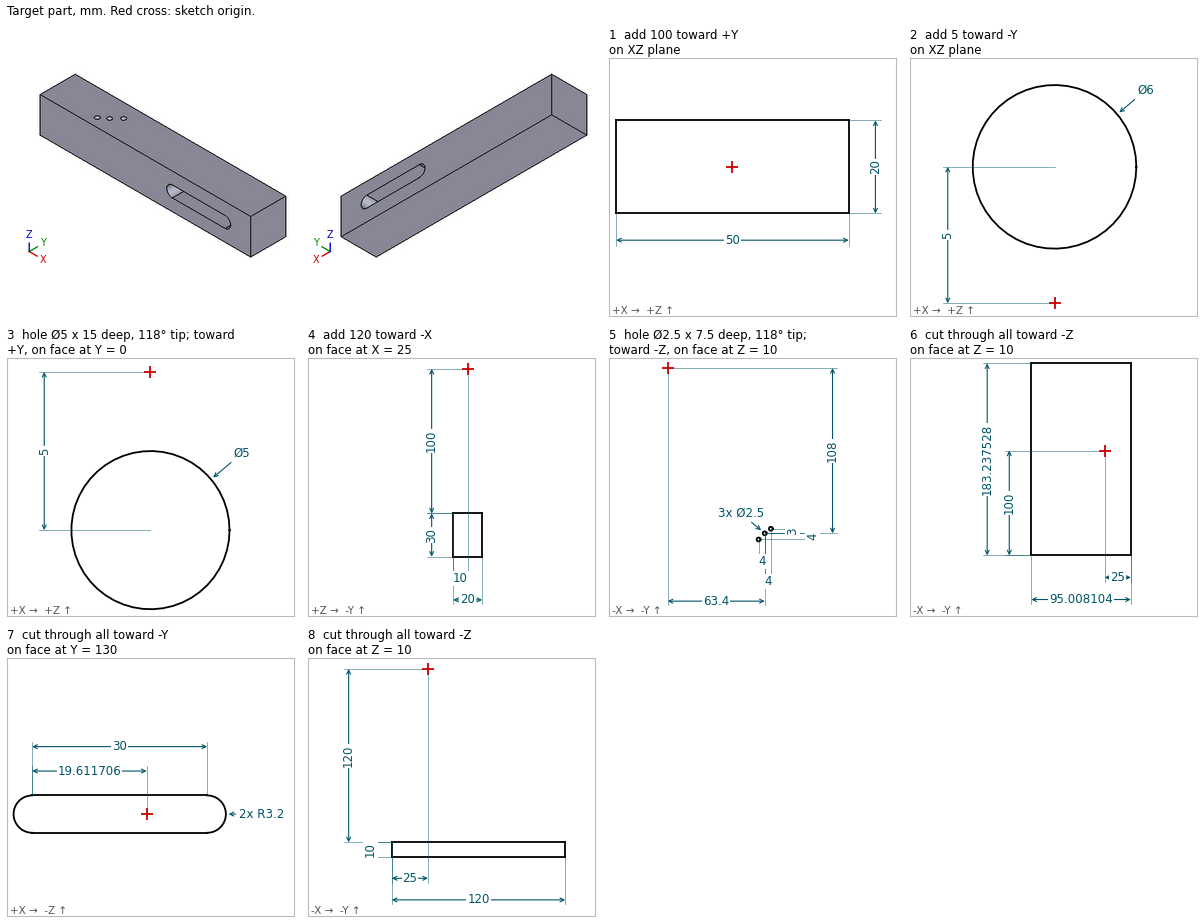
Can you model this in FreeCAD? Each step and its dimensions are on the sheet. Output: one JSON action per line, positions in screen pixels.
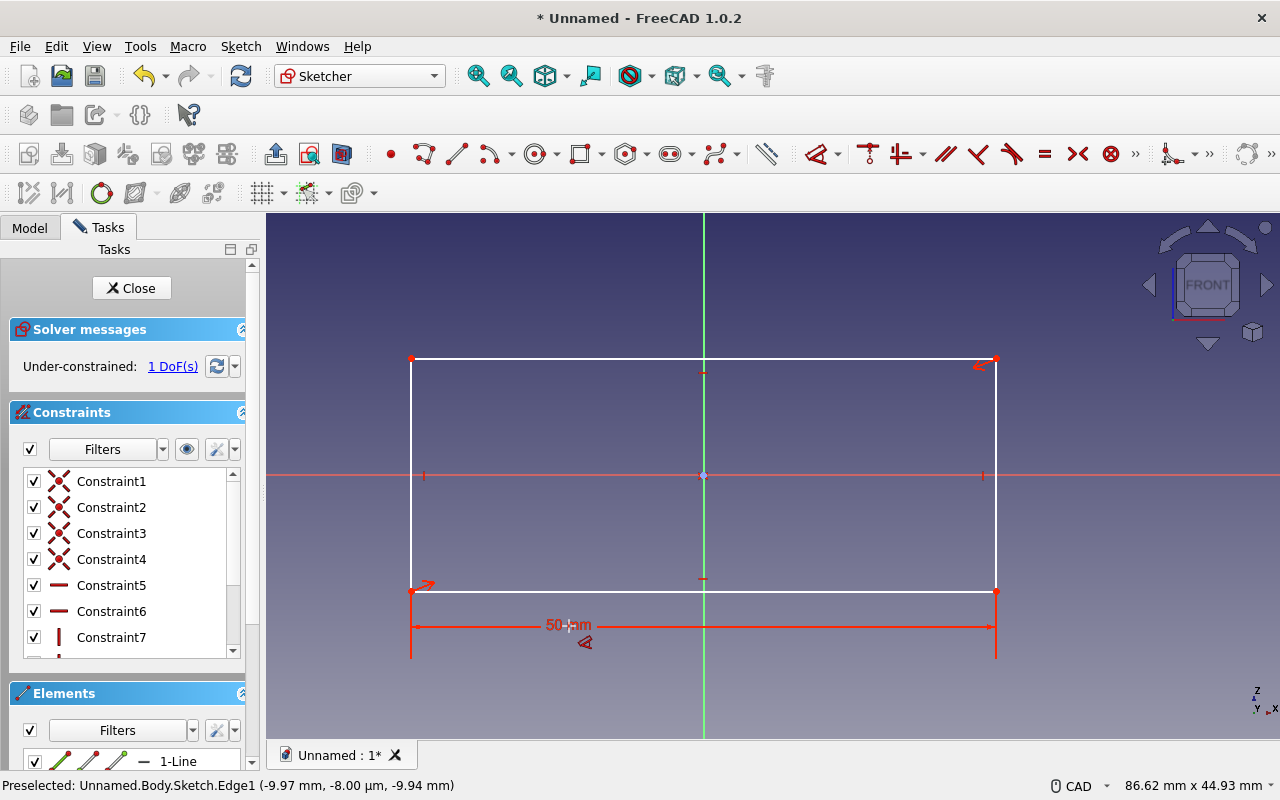
{"action": "left_click", "coordinate": [996, 522]}
{"action": "left_click", "coordinate": [1030, 422]}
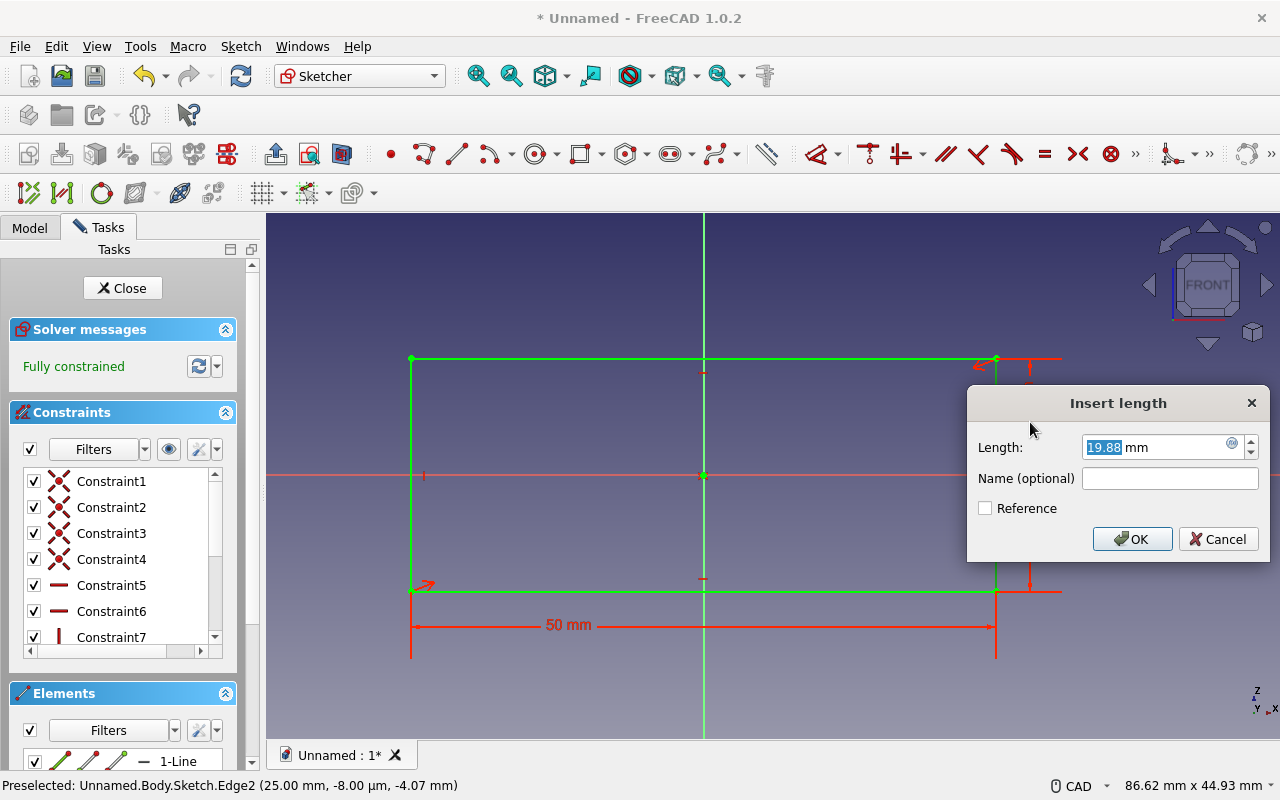
{"action": "type", "text": "20"}
{"action": "key", "text": "Return"}
{"action": "key", "text": "Escape"}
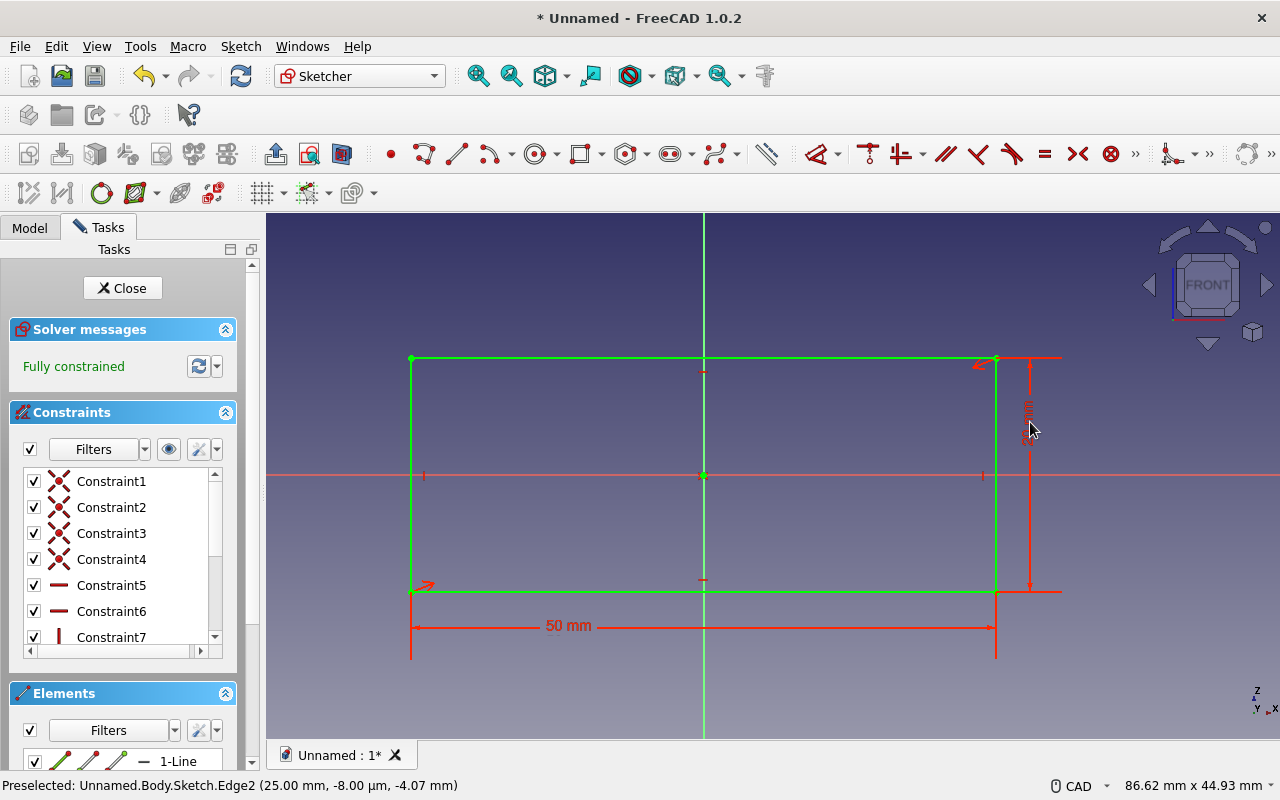
{"action": "left_click", "coordinate": [123, 288]}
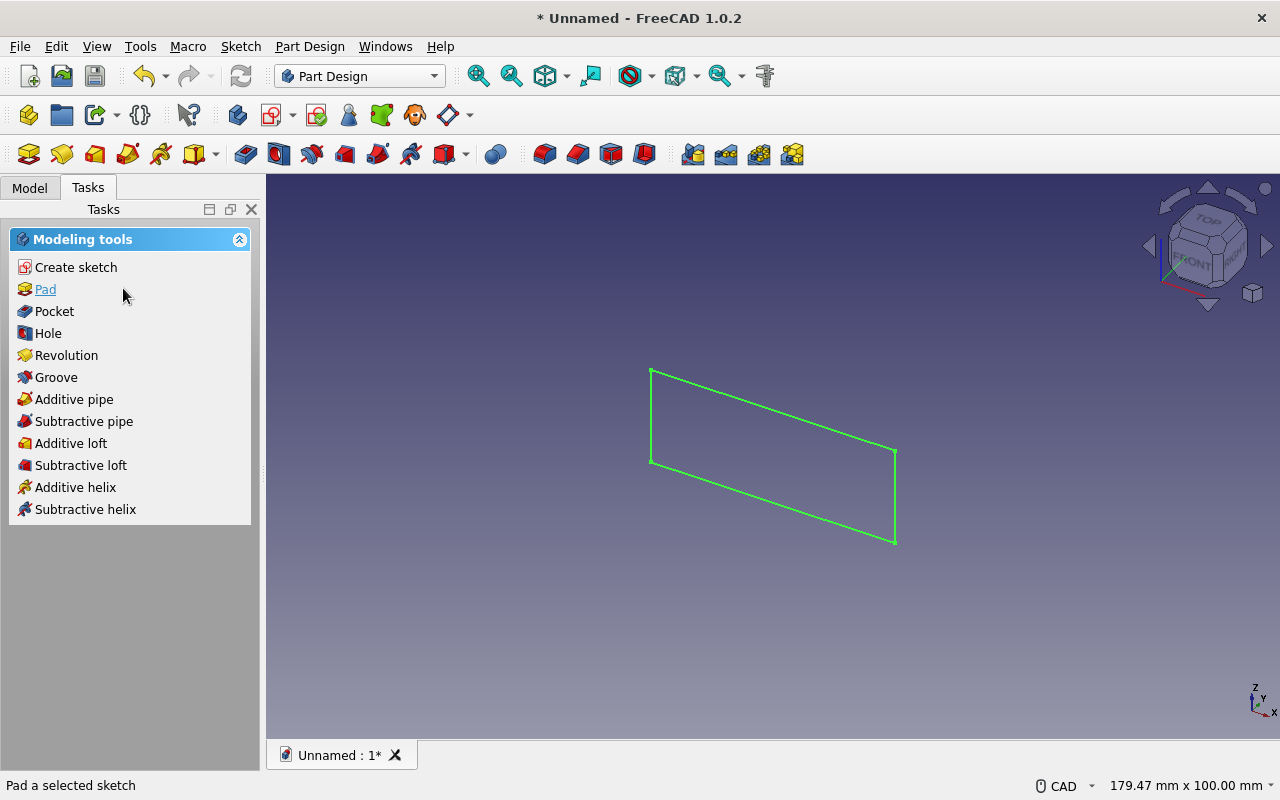
{"action": "left_click", "coordinate": [29, 154]}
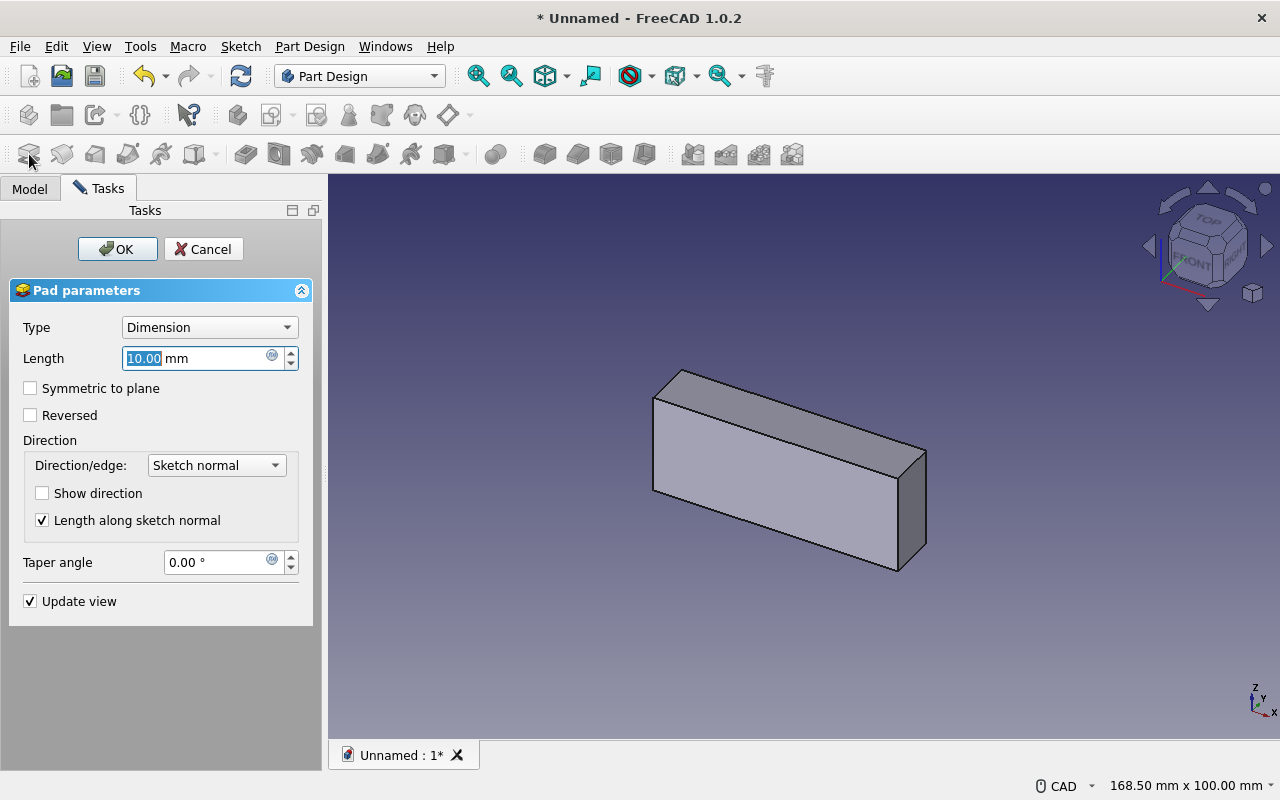
{"action": "type", "text": "100"}
{"action": "key", "text": "Tab"}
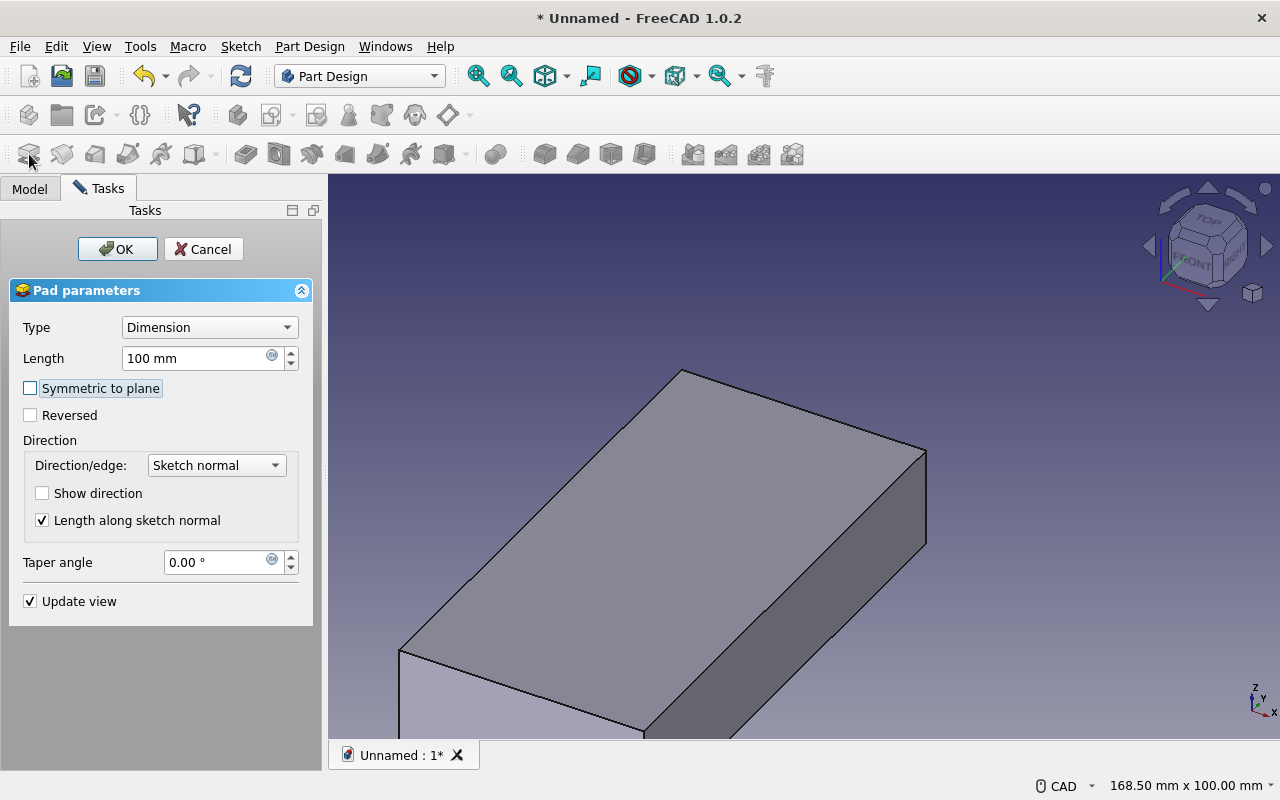
{"action": "left_click", "coordinate": [31, 415]}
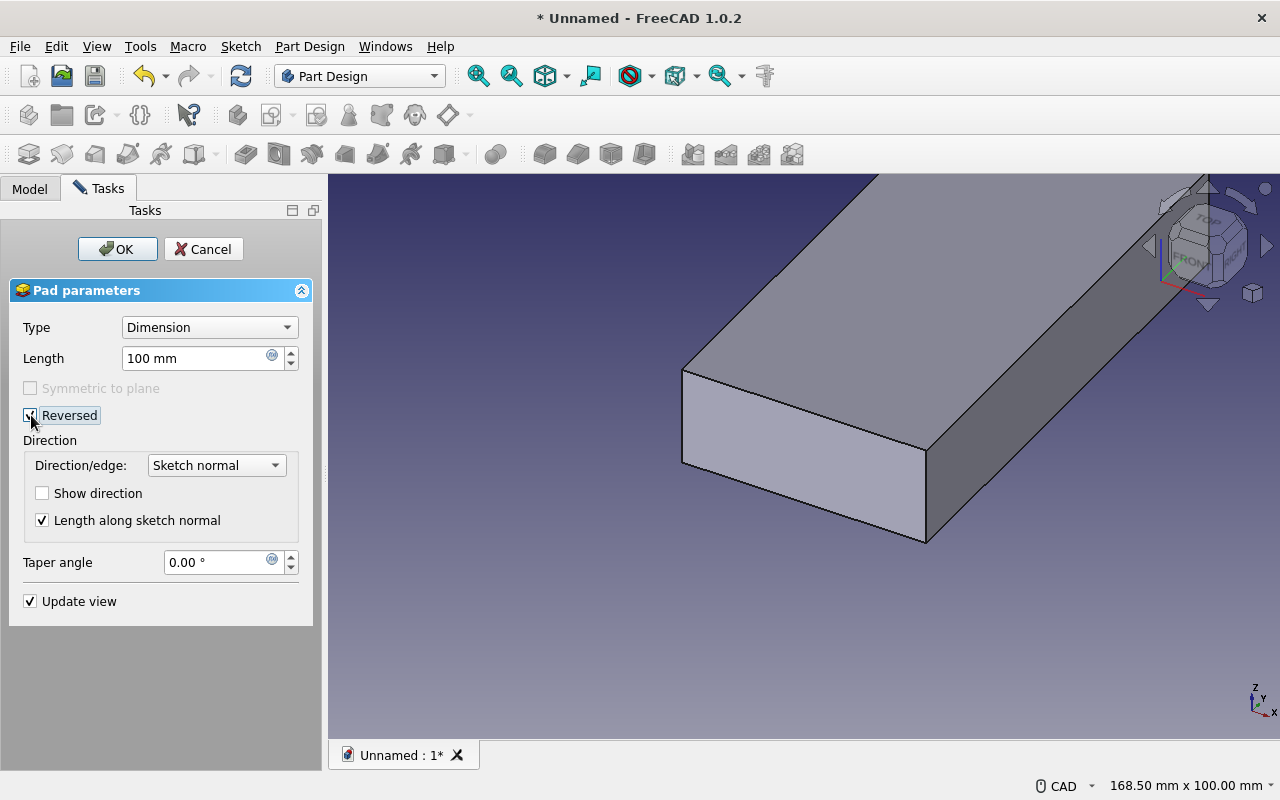
{"action": "left_click", "coordinate": [118, 249]}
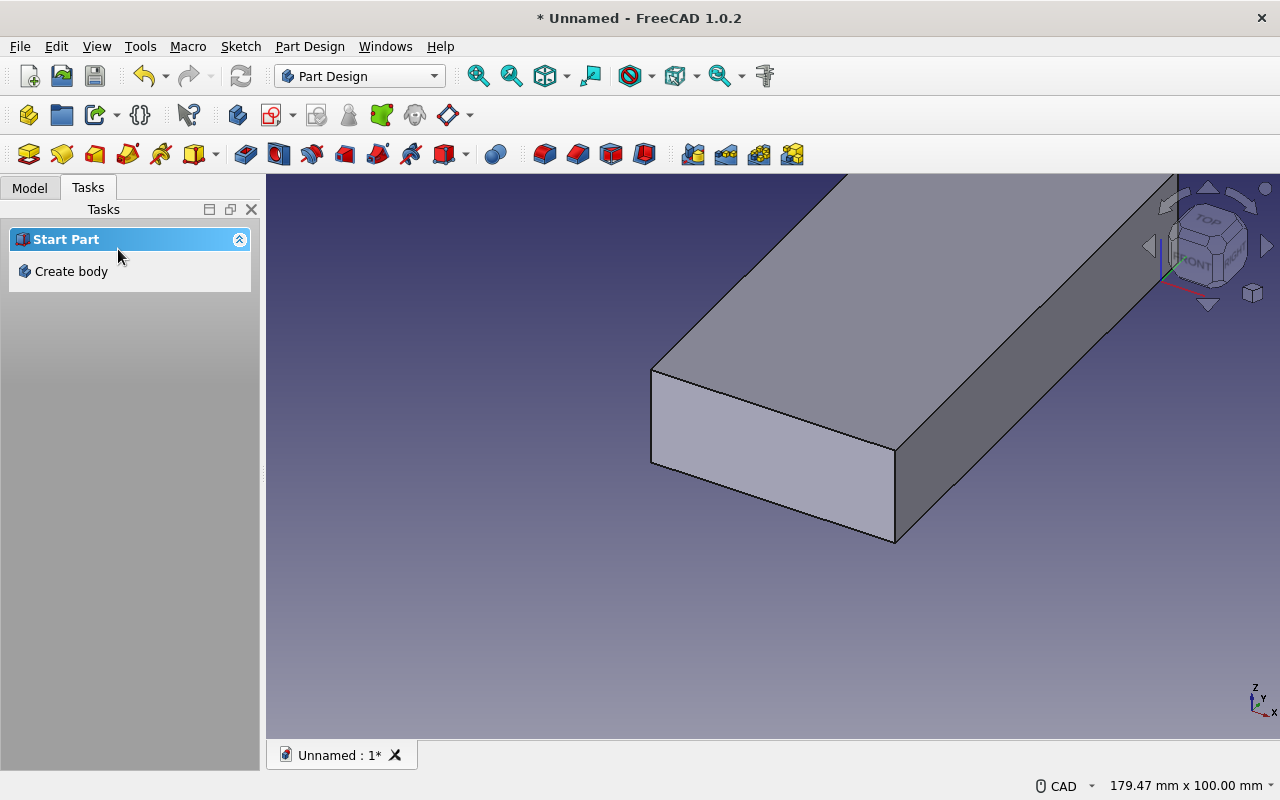
{"action": "left_click", "coordinate": [479, 76]}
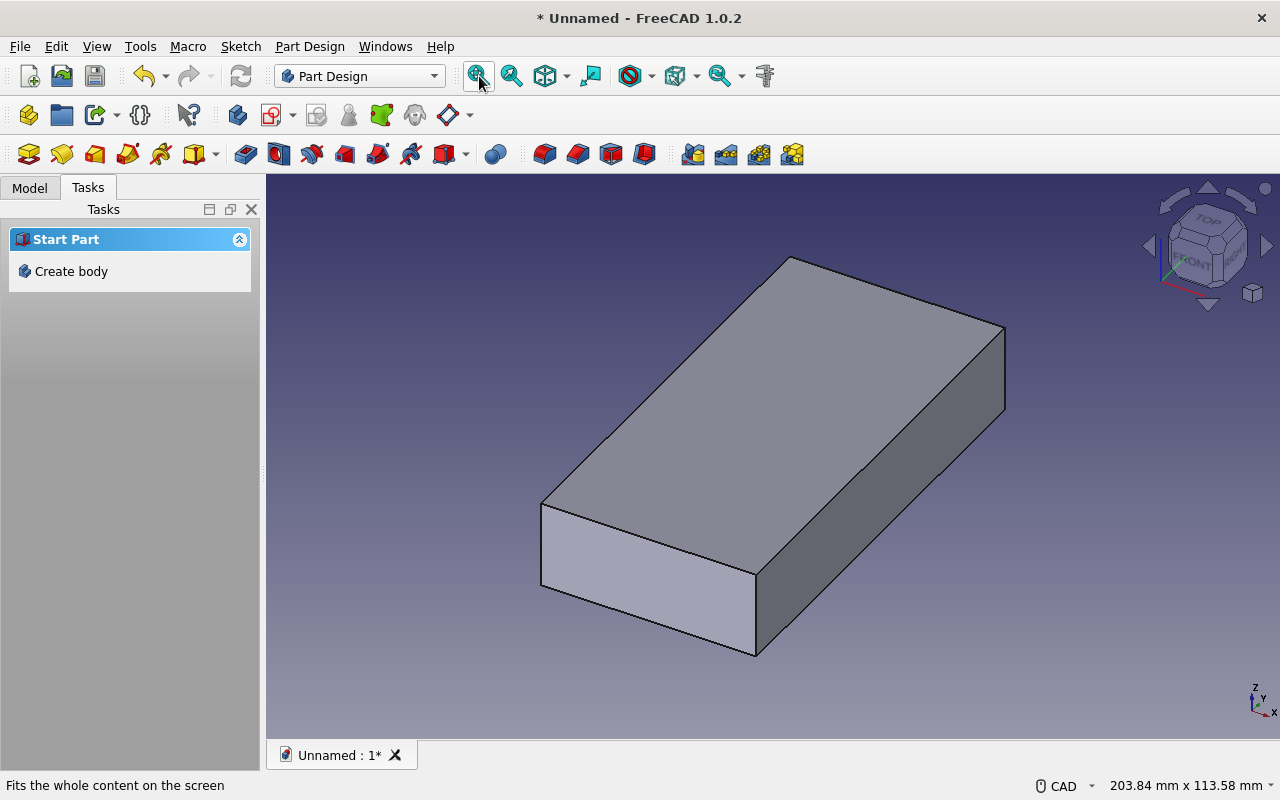
{"action": "left_click", "coordinate": [270, 116]}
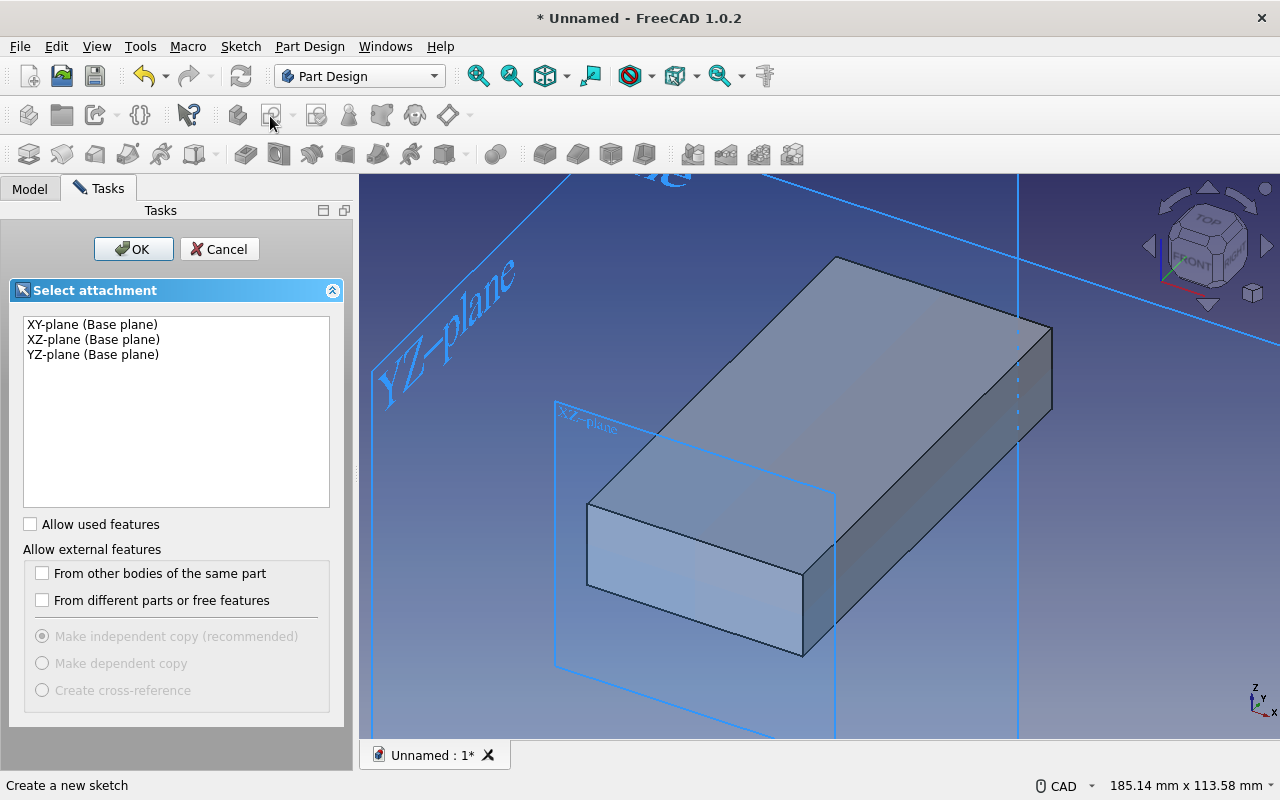
{"action": "left_click", "coordinate": [84, 340]}